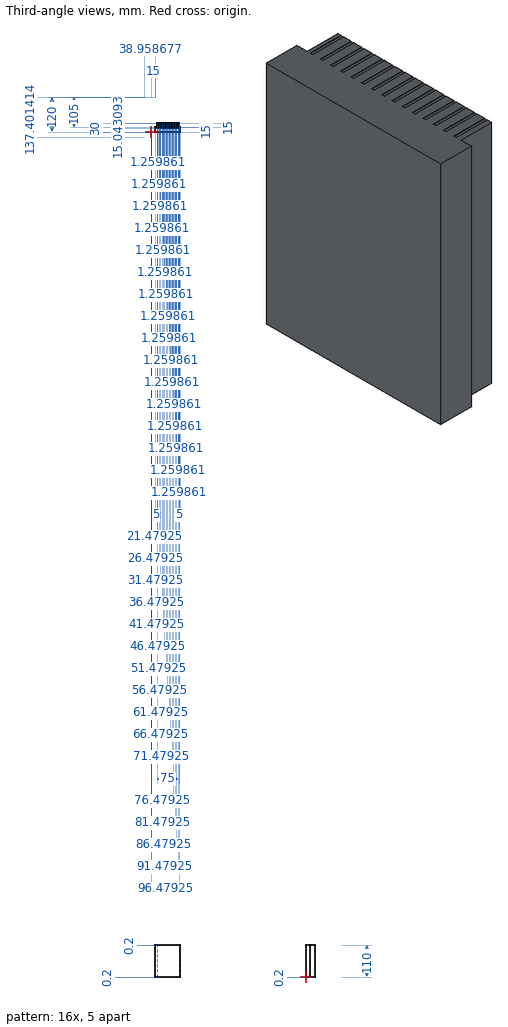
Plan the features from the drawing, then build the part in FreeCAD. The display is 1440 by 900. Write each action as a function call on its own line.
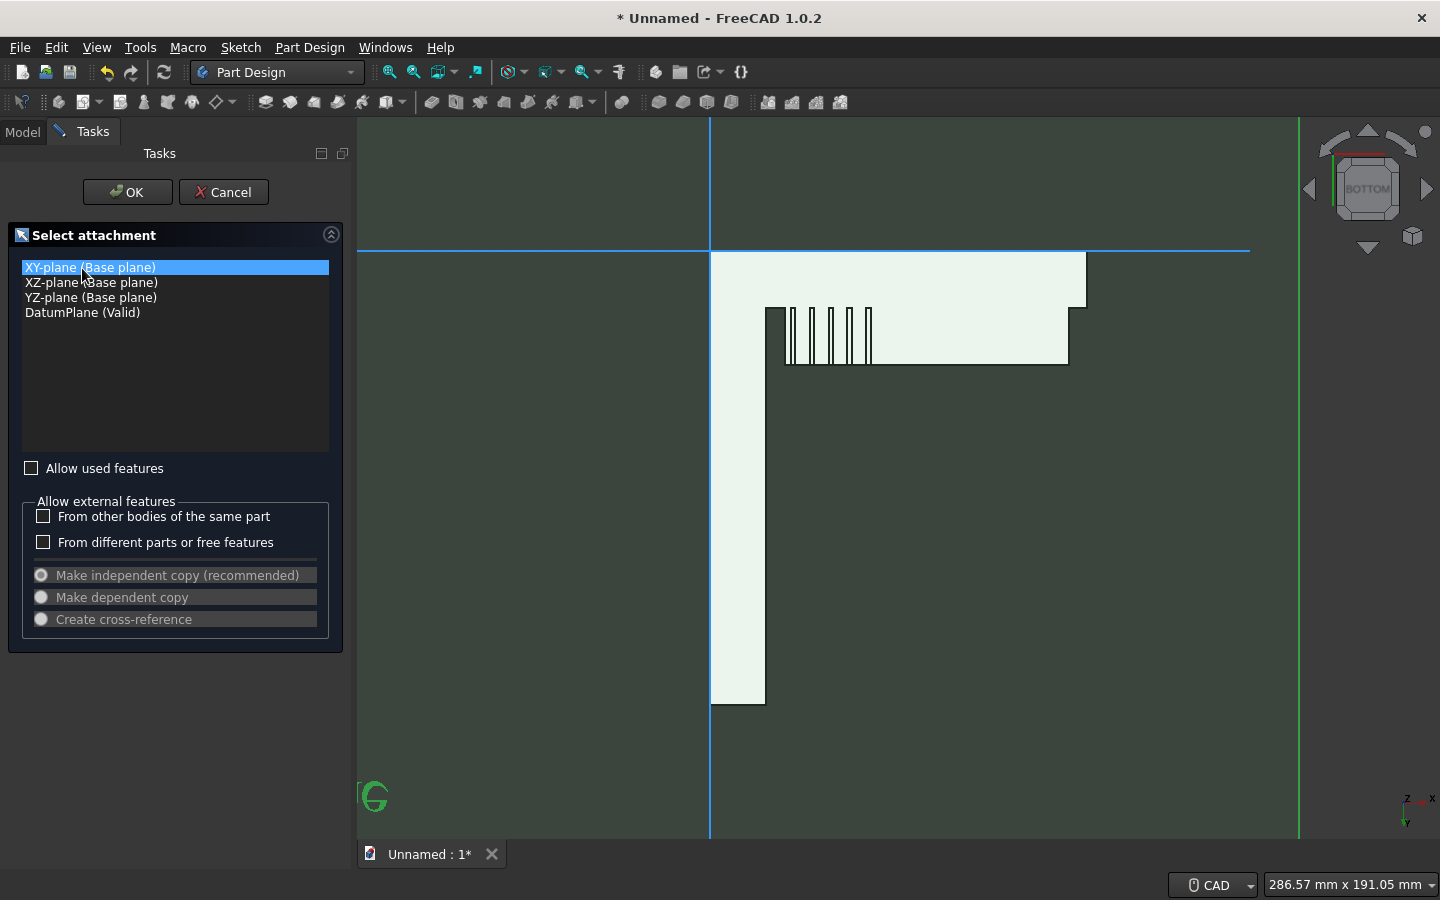
click(128, 192)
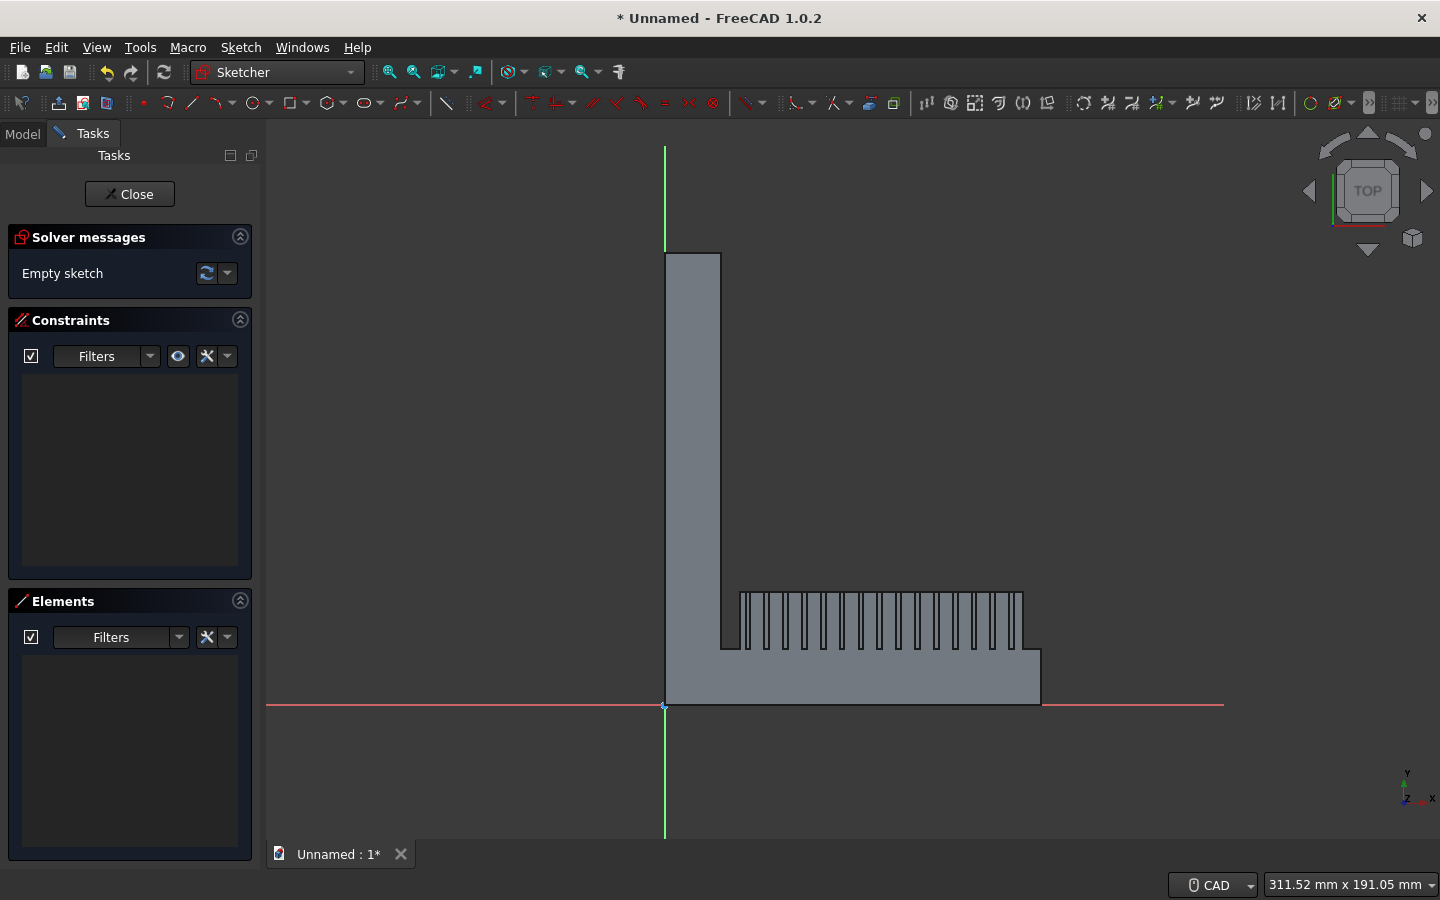
click(108, 104)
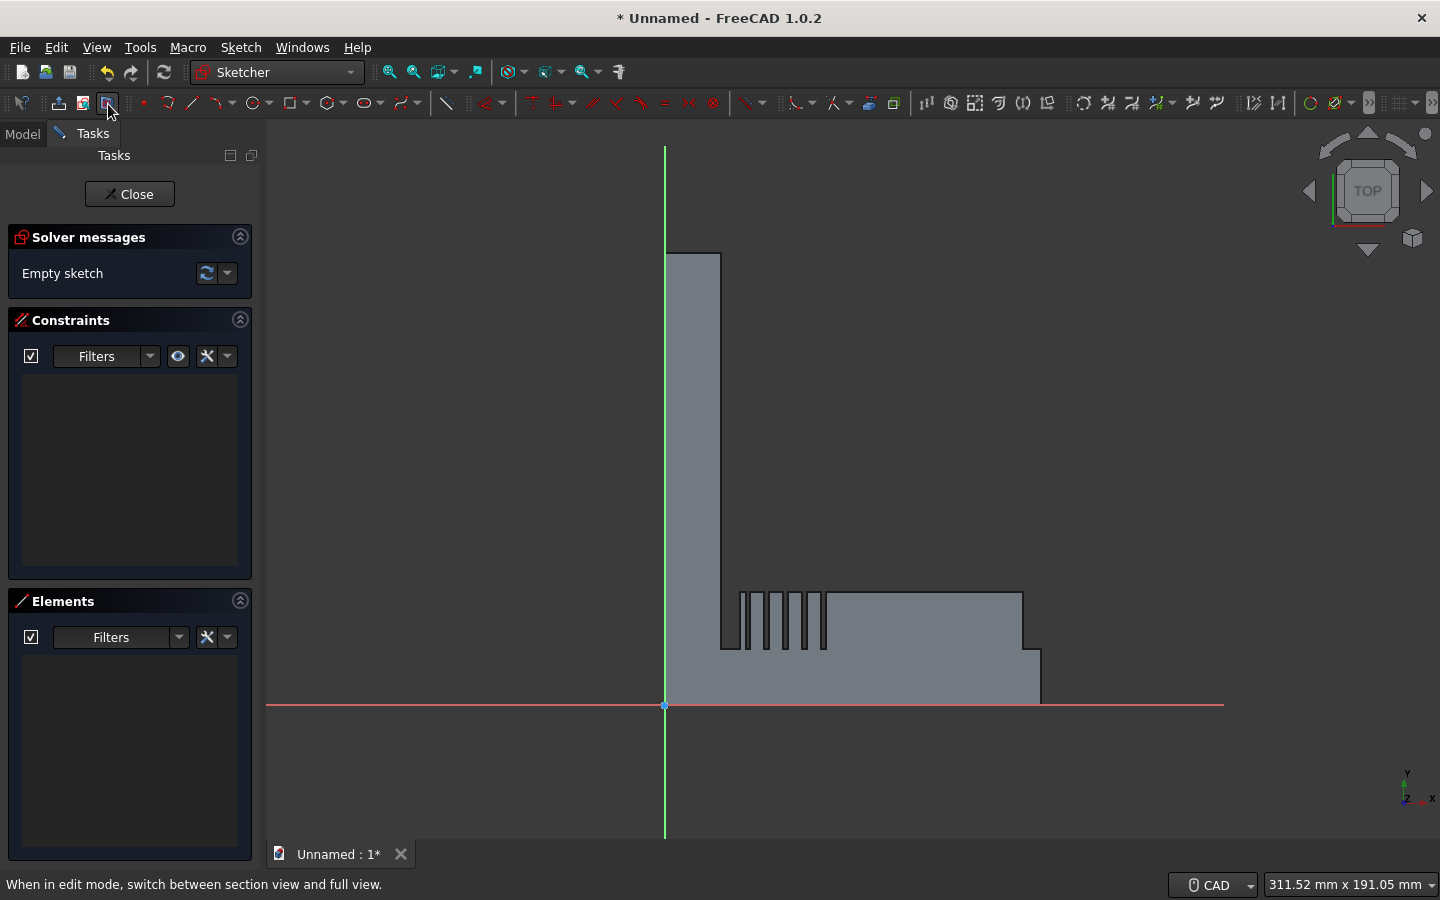
scroll(849, 638, up, 11)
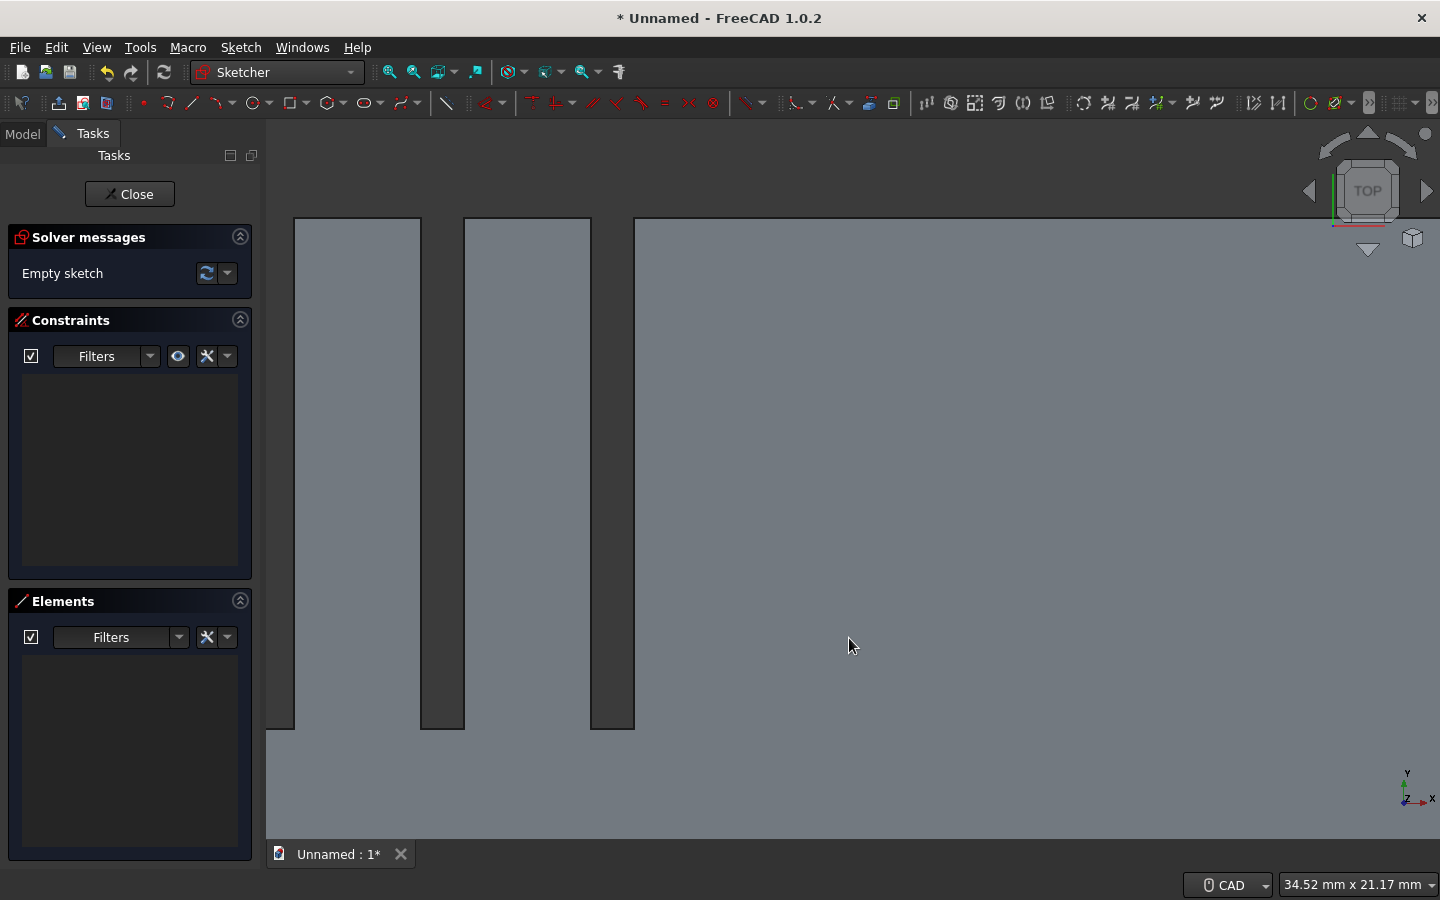
click(290, 104)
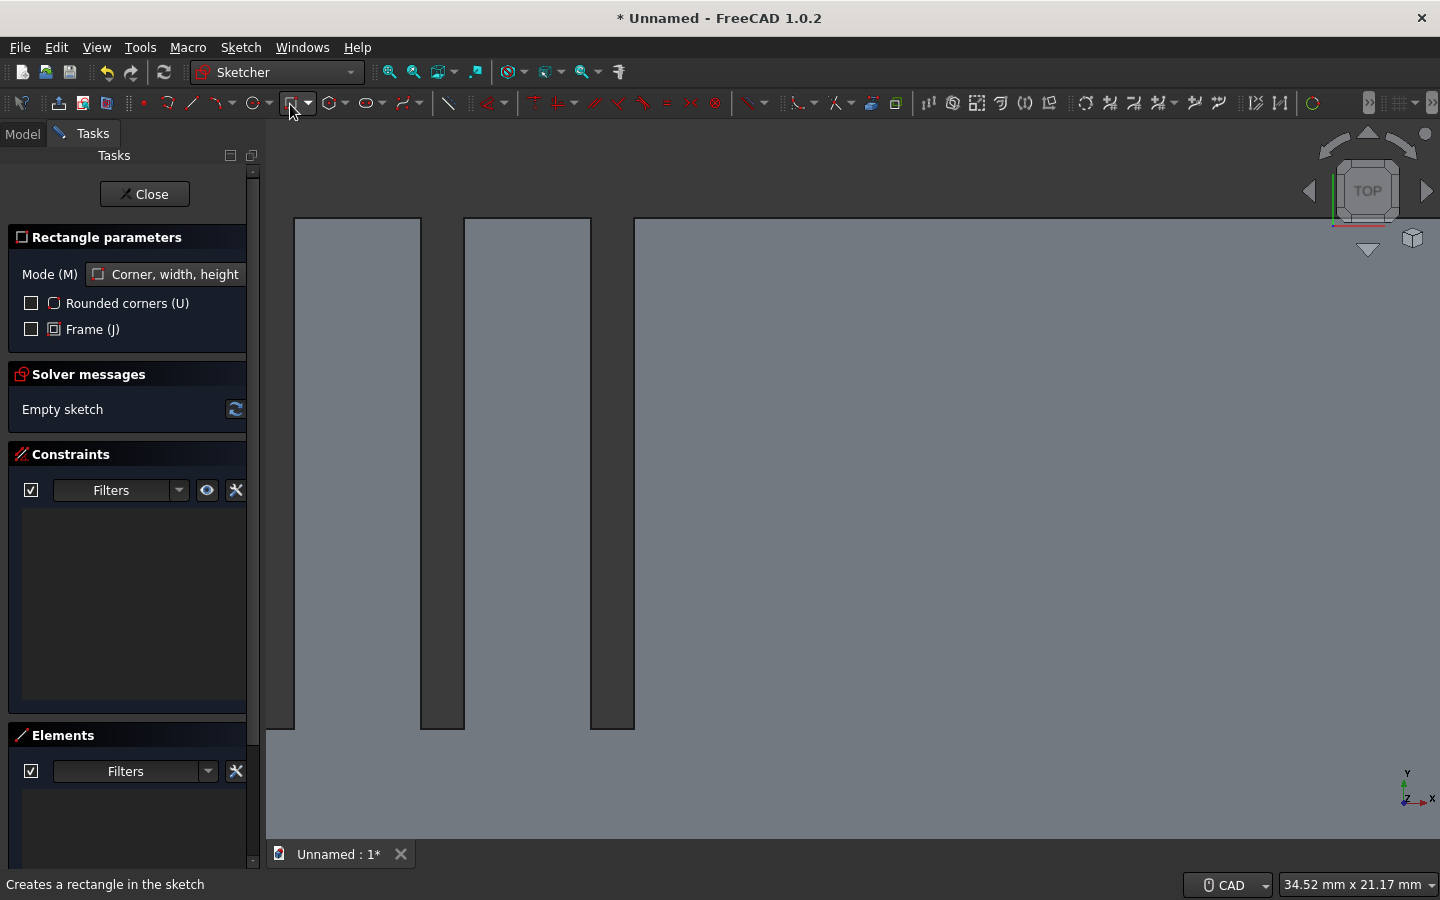
click(761, 218)
click(804, 729)
key(Escape)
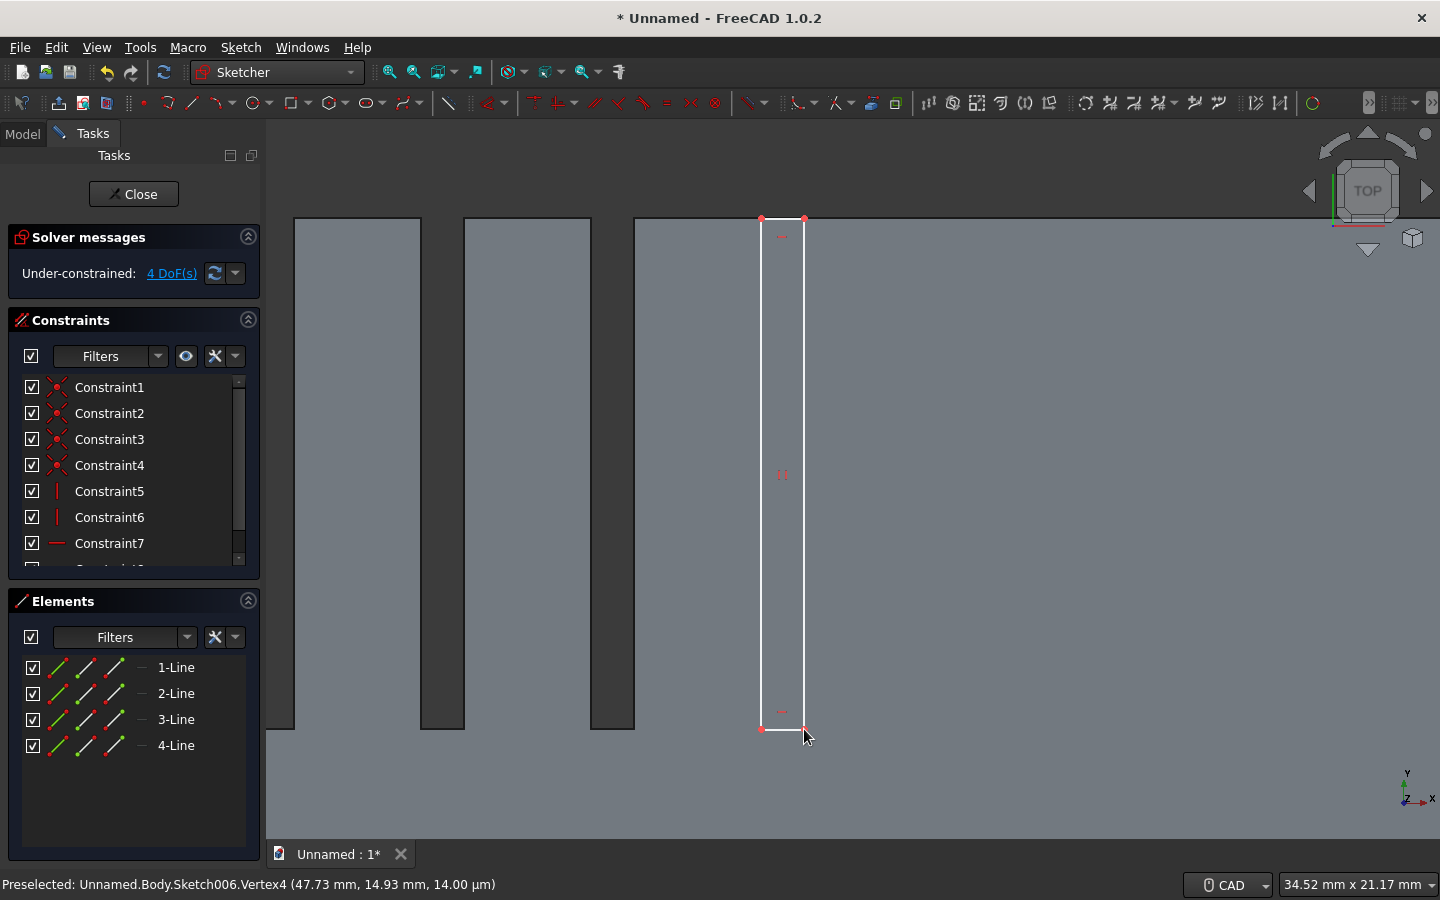
click(488, 104)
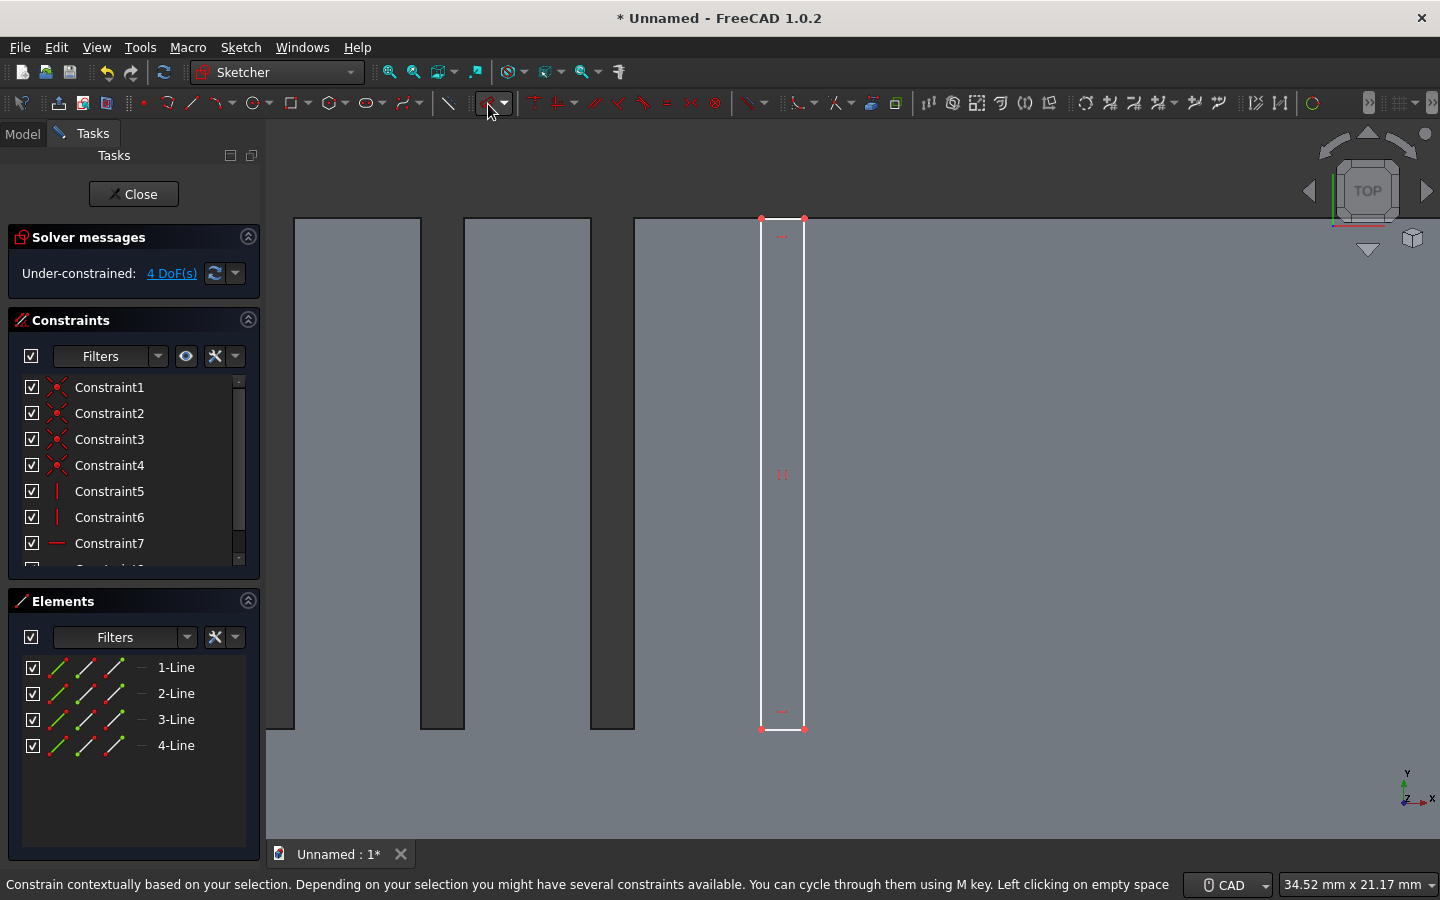
click(761, 219)
click(819, 515)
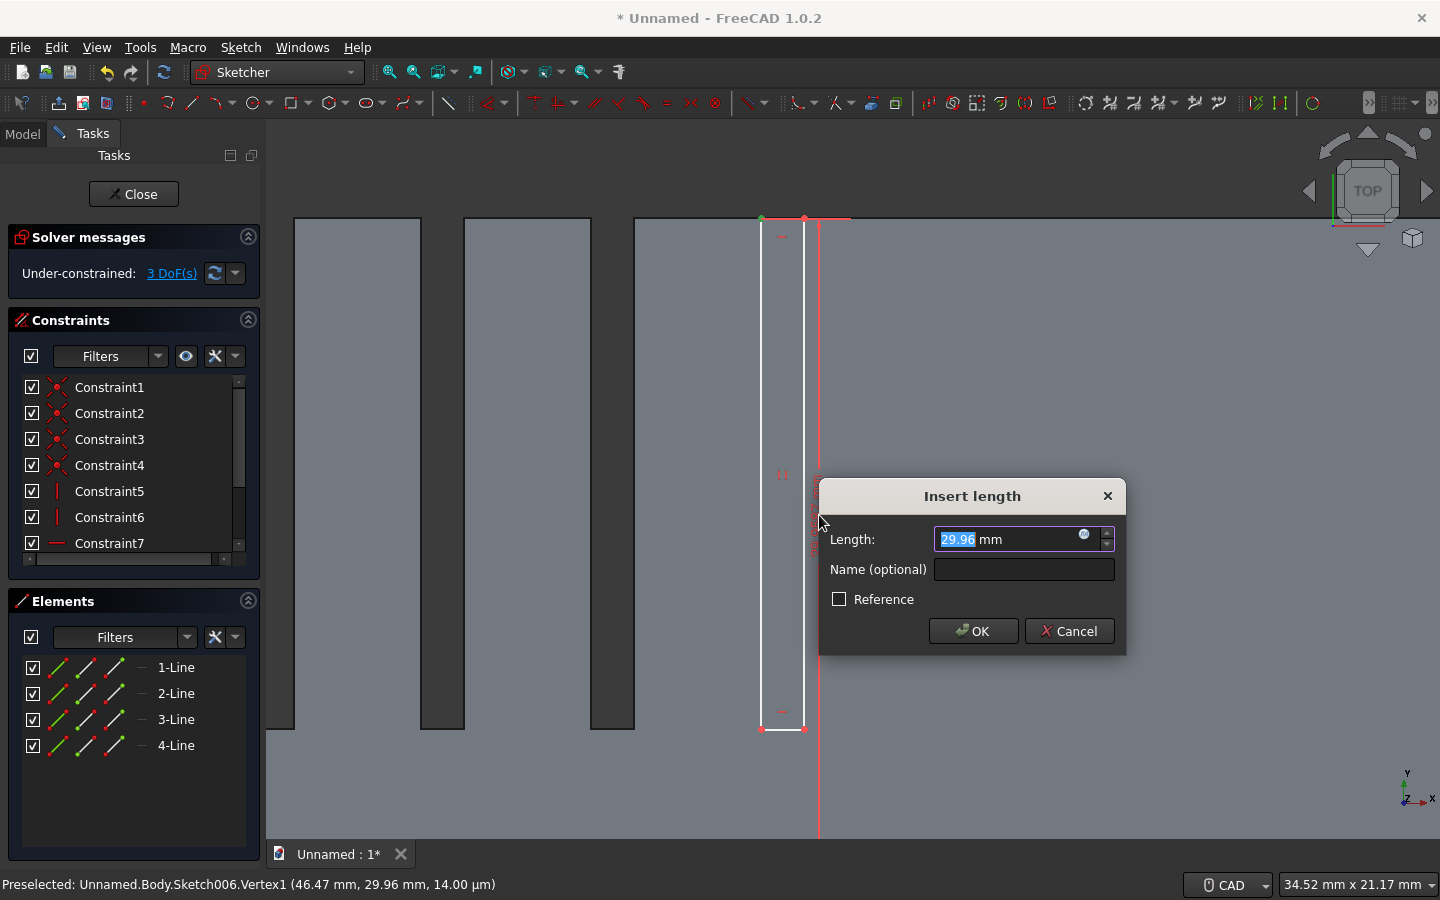
text(30)
key(Return)